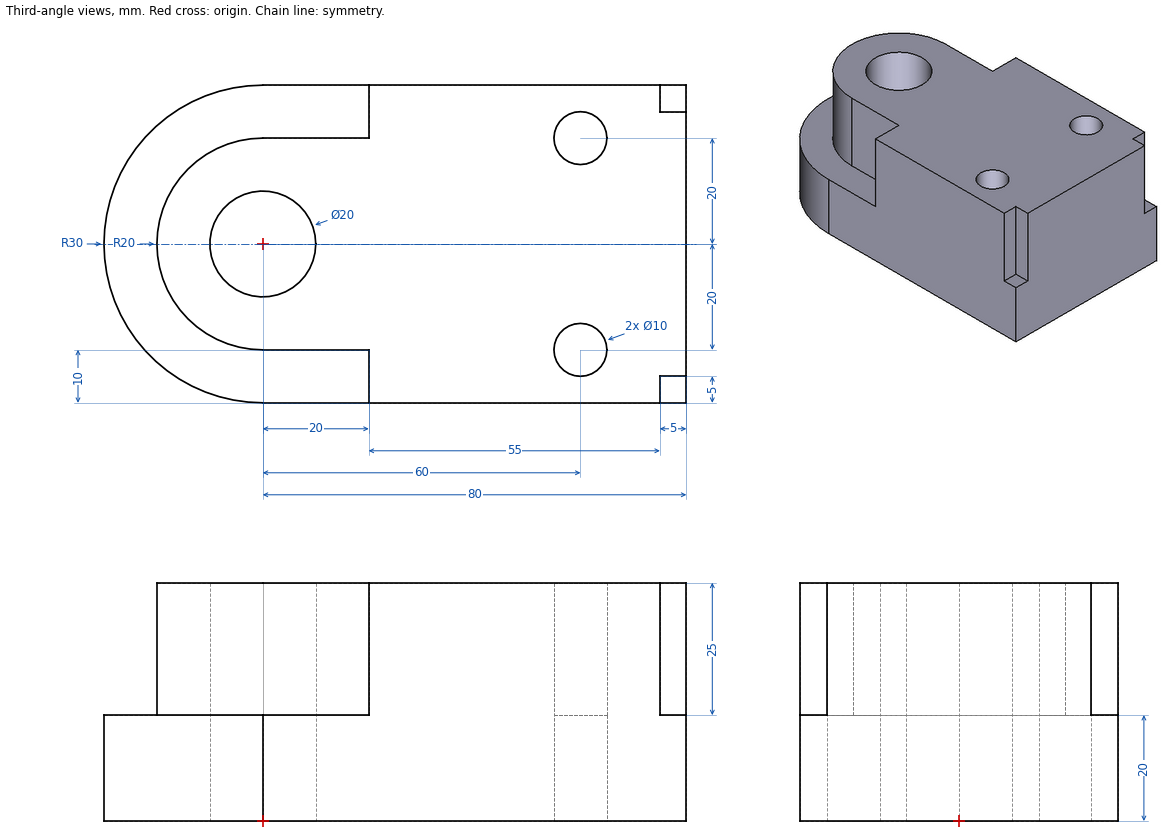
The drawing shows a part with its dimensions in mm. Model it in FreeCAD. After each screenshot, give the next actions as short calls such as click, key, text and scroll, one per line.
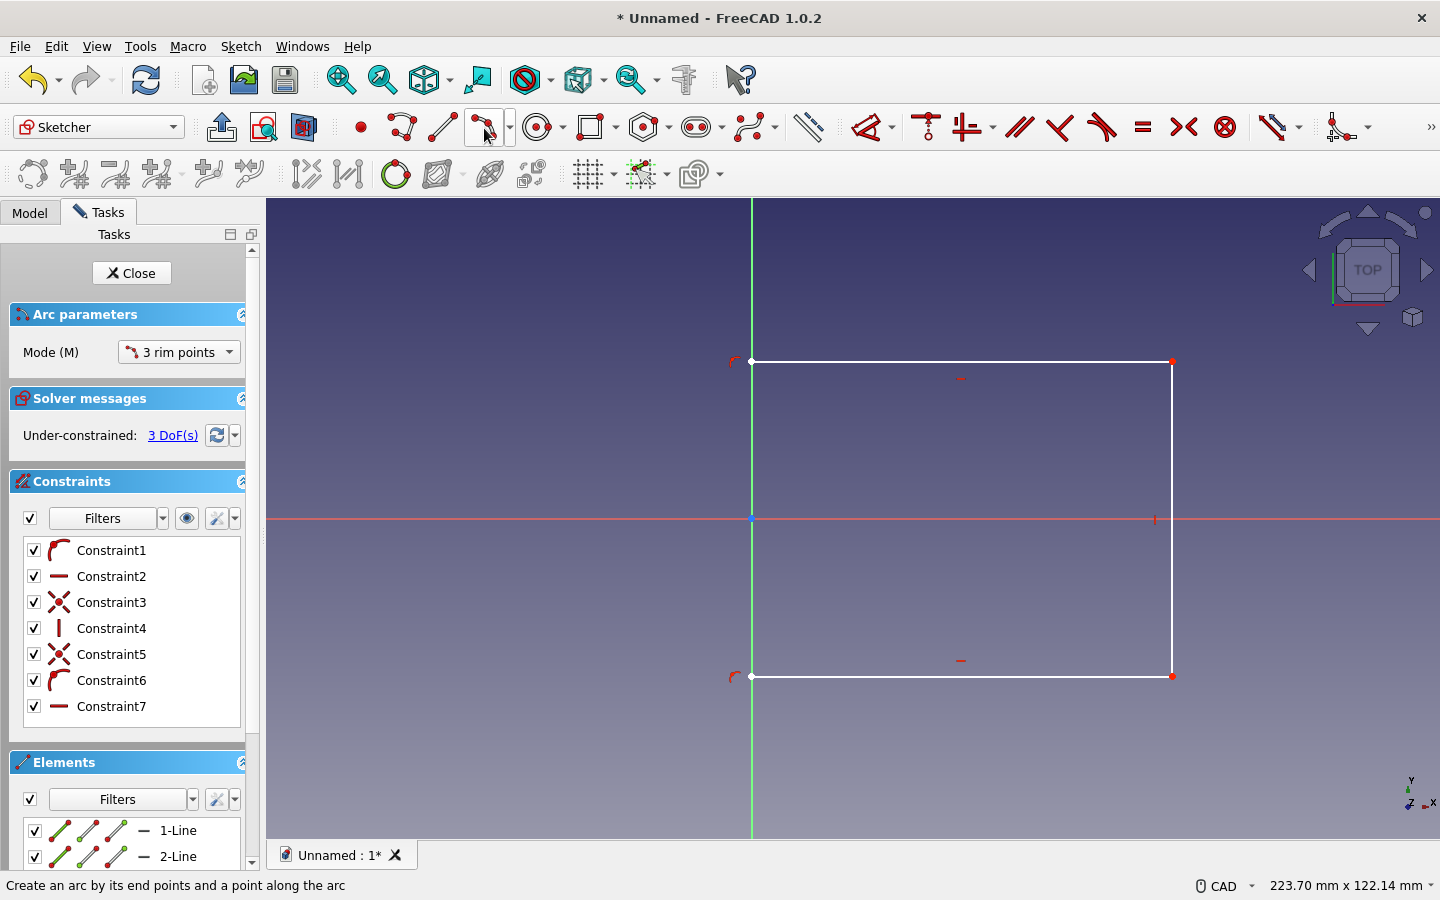
click(752, 362)
click(752, 677)
click(602, 470)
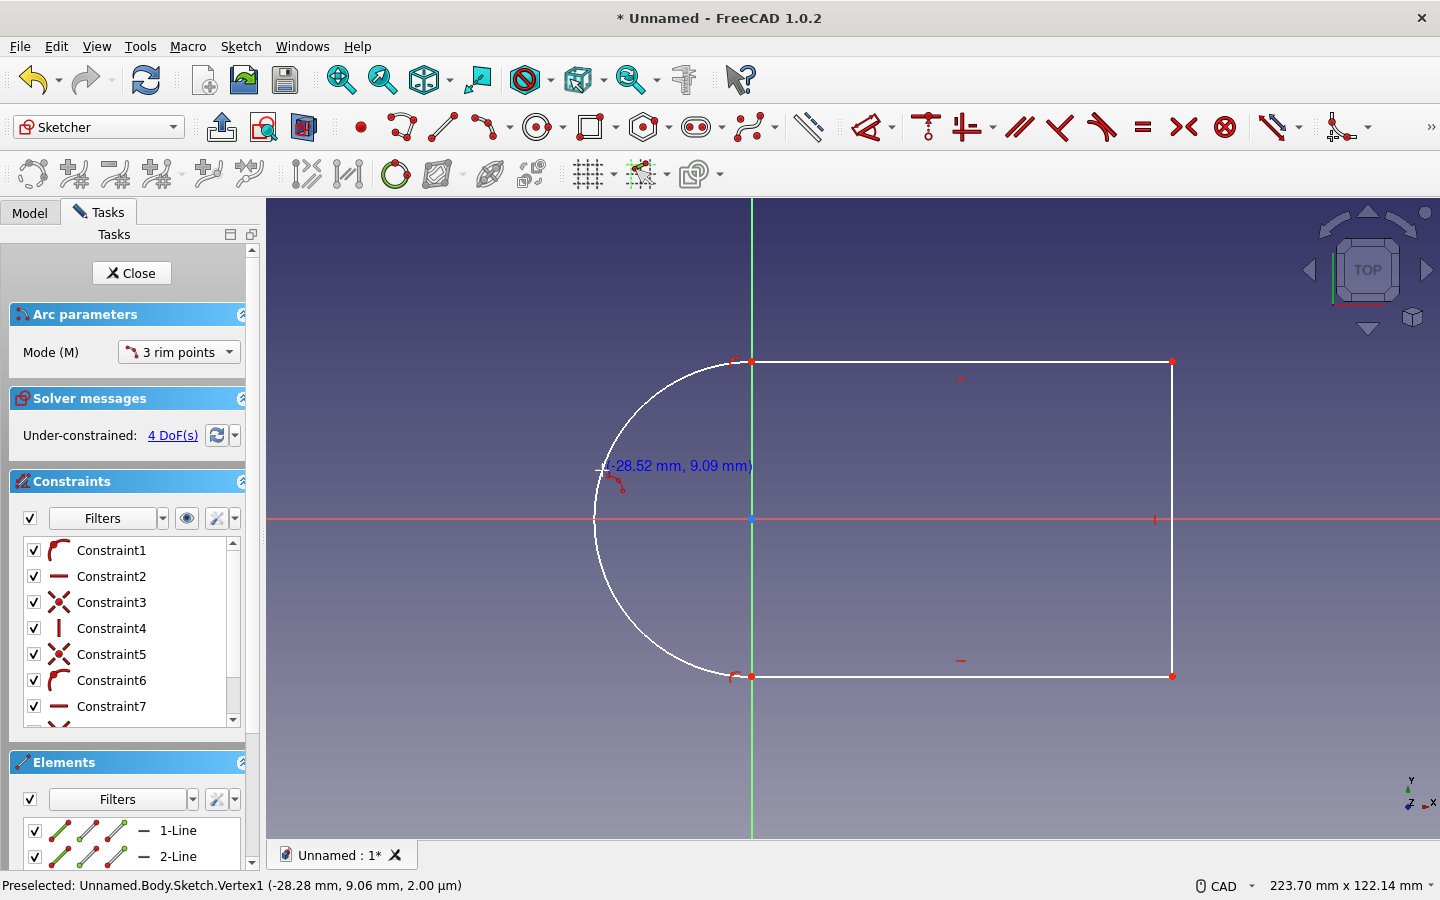
click(536, 128)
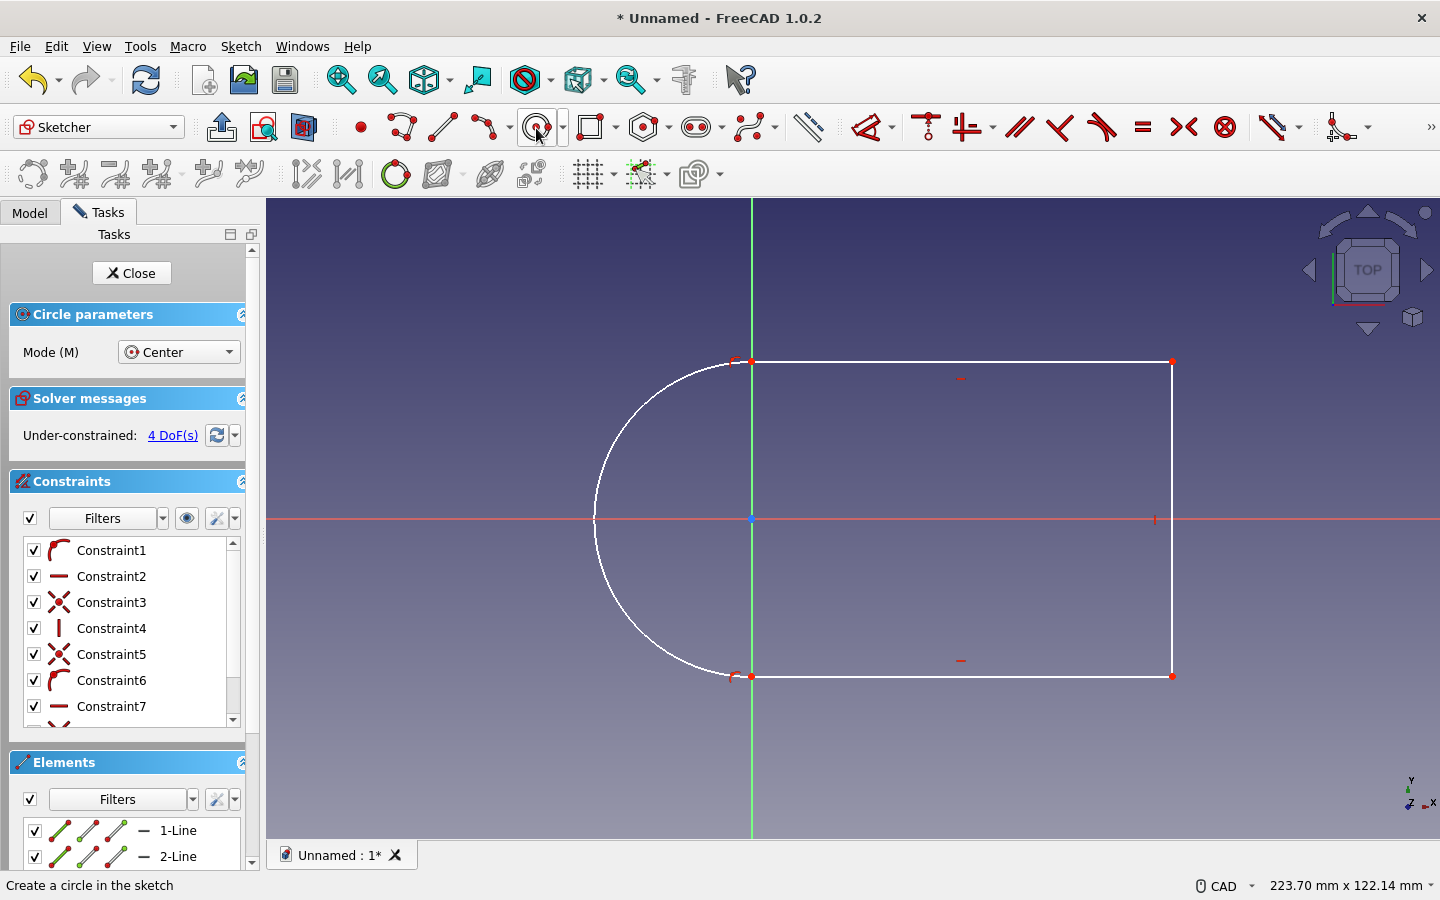
click(752, 519)
move(789, 482)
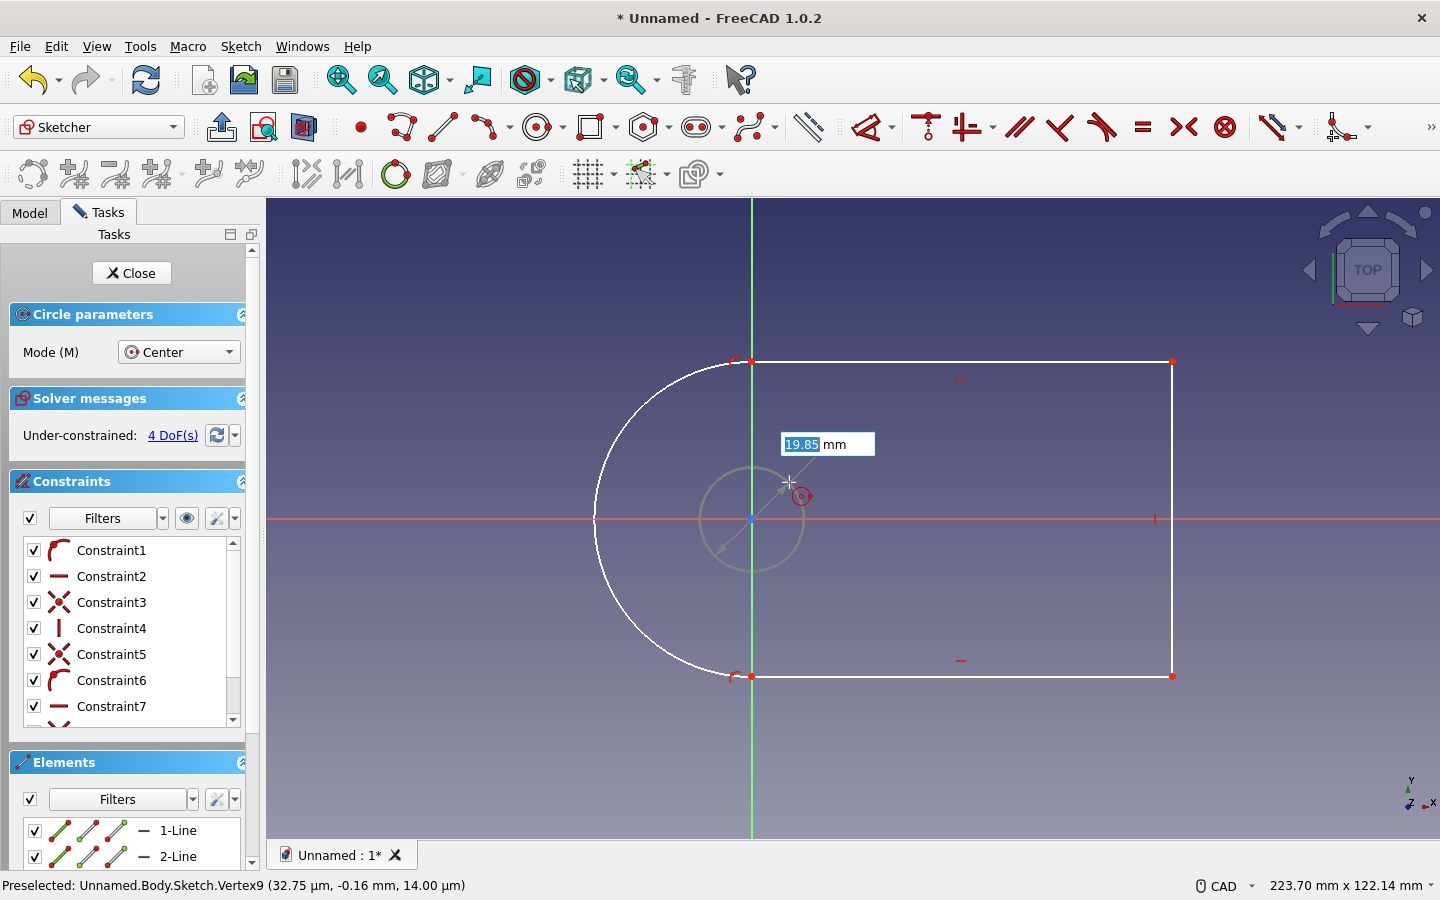
text(20)
key(Return)
key(Escape)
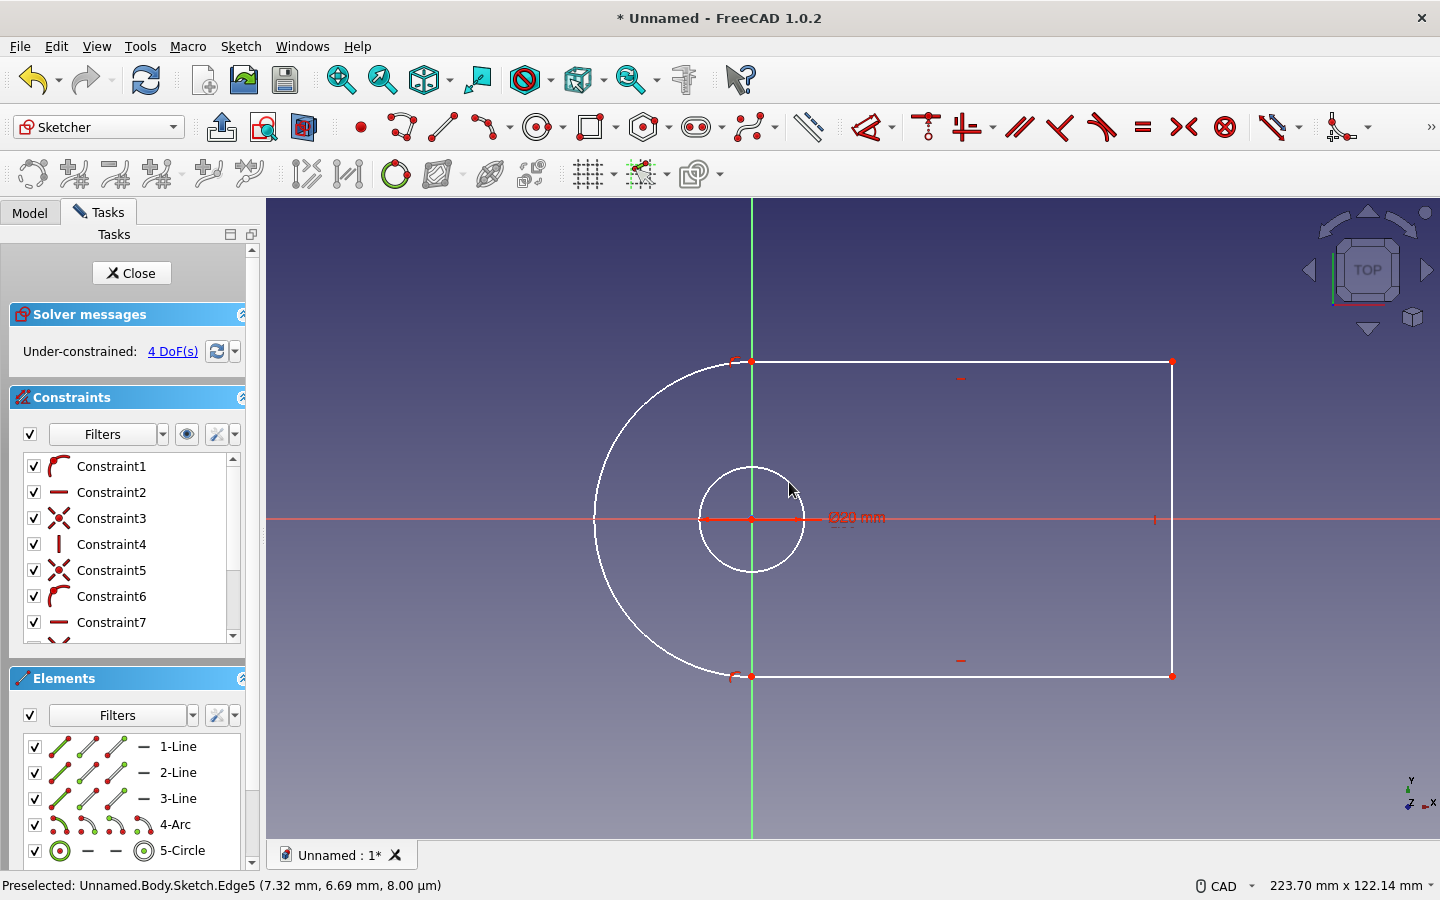
drag(742, 509, 762, 530)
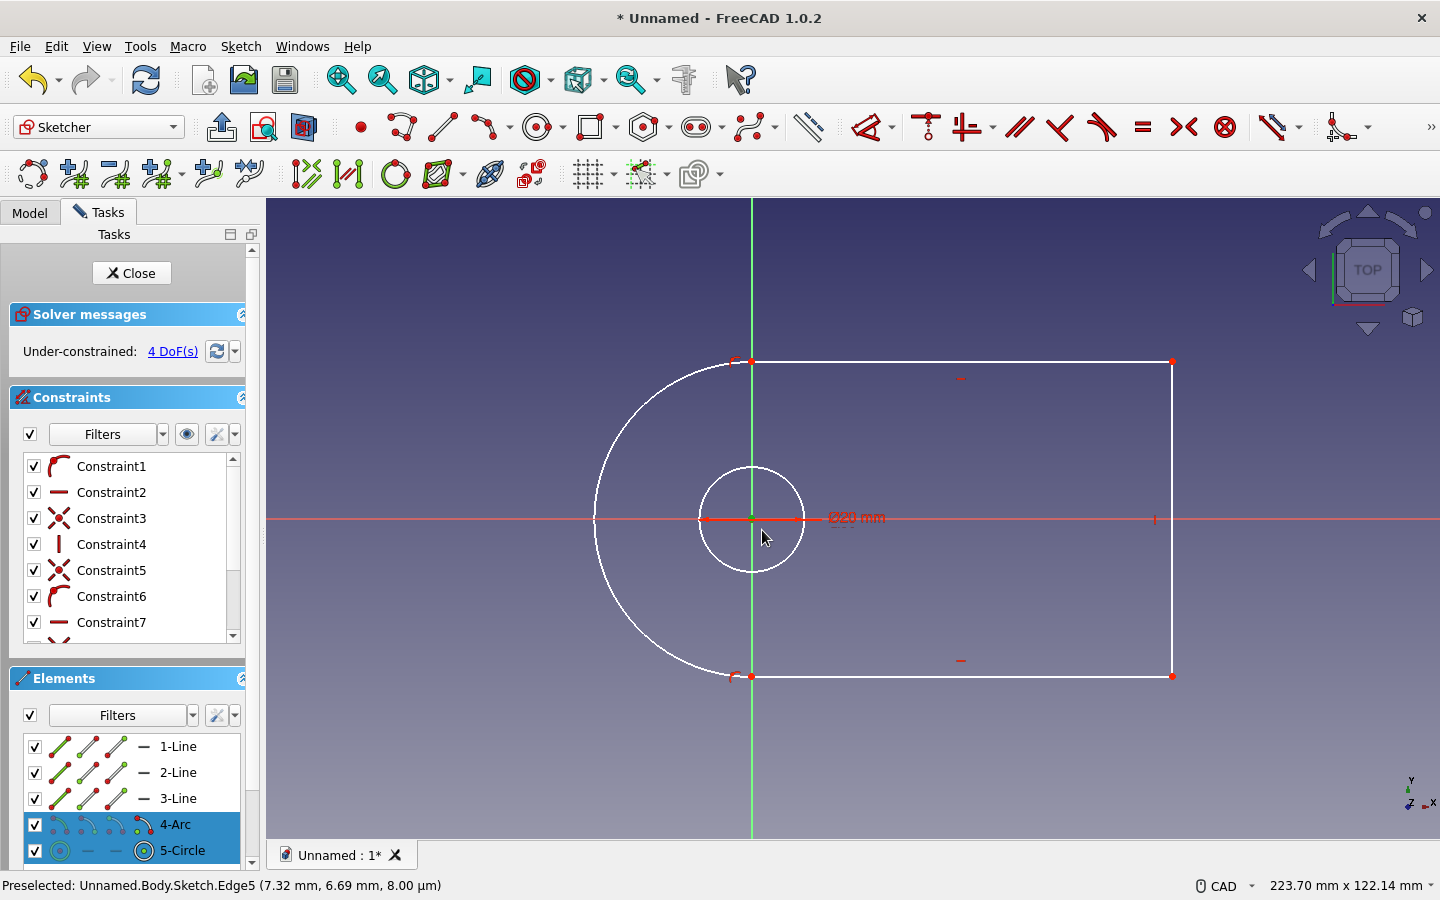
key(c)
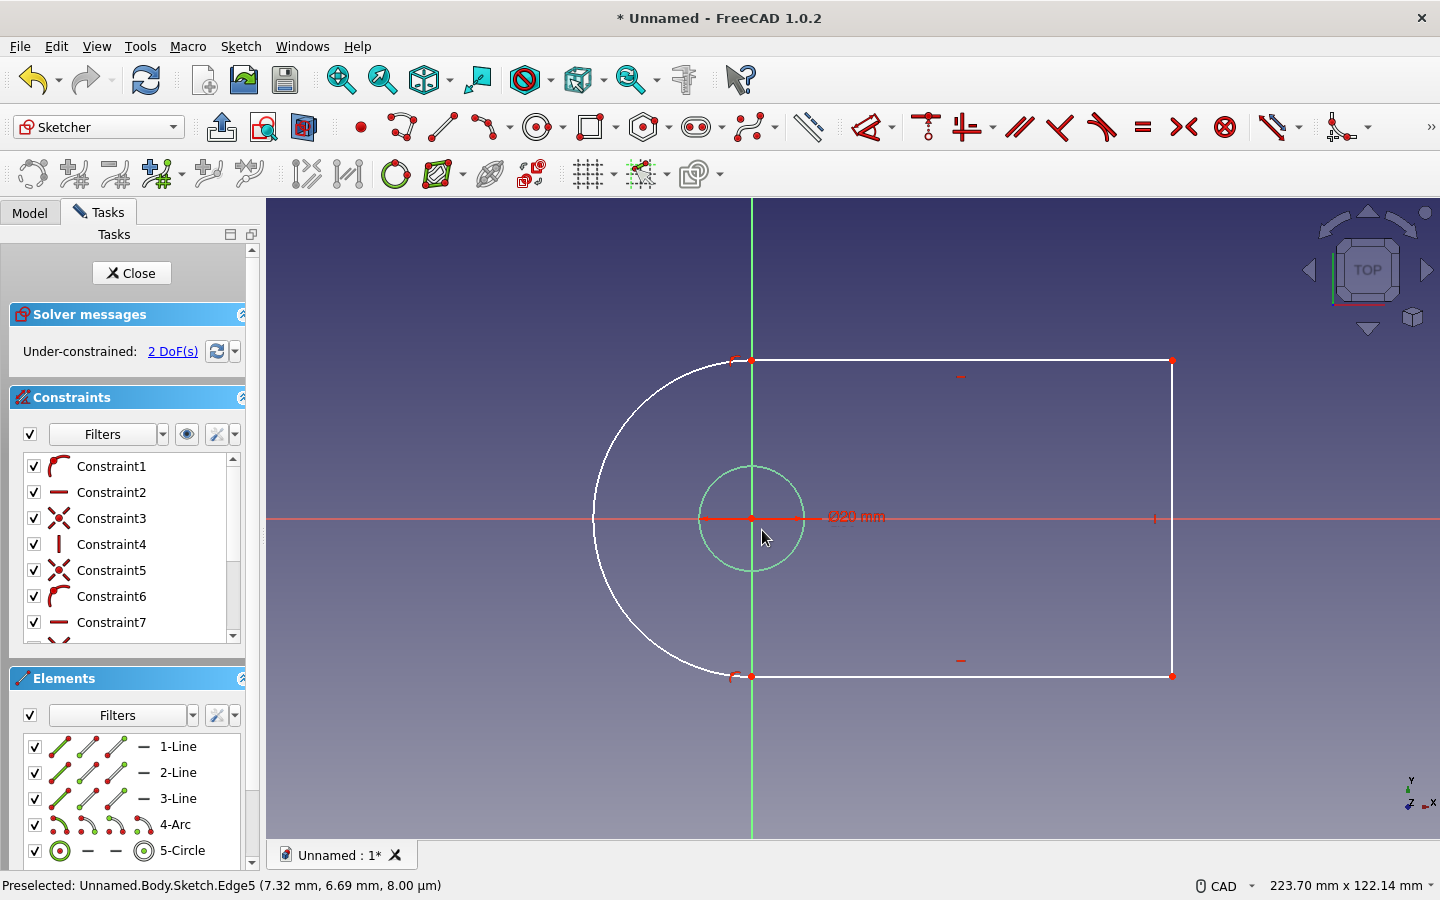
click(866, 128)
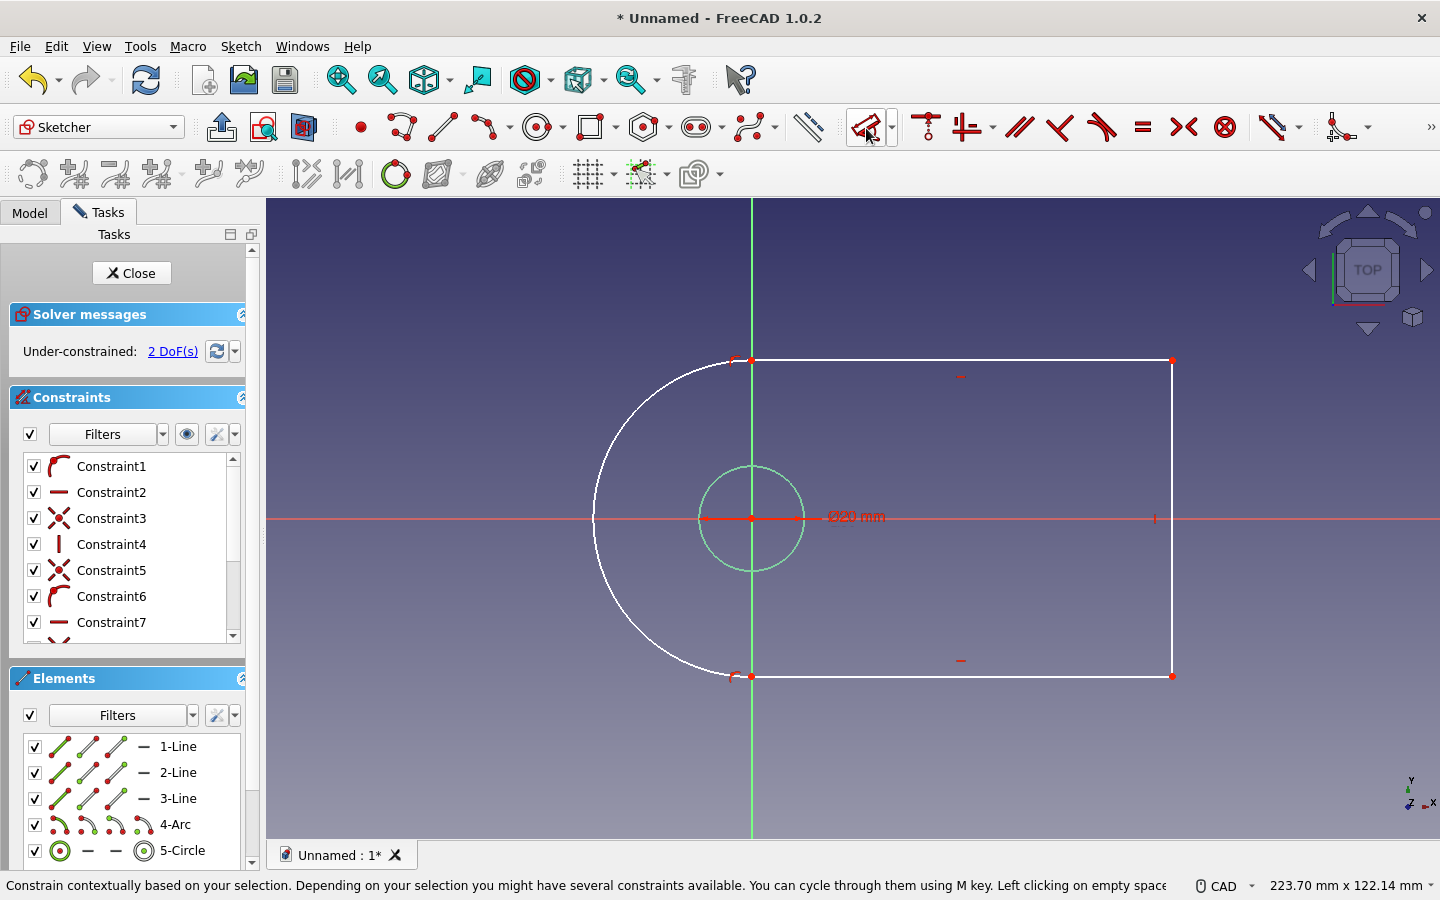
click(624, 426)
click(598, 407)